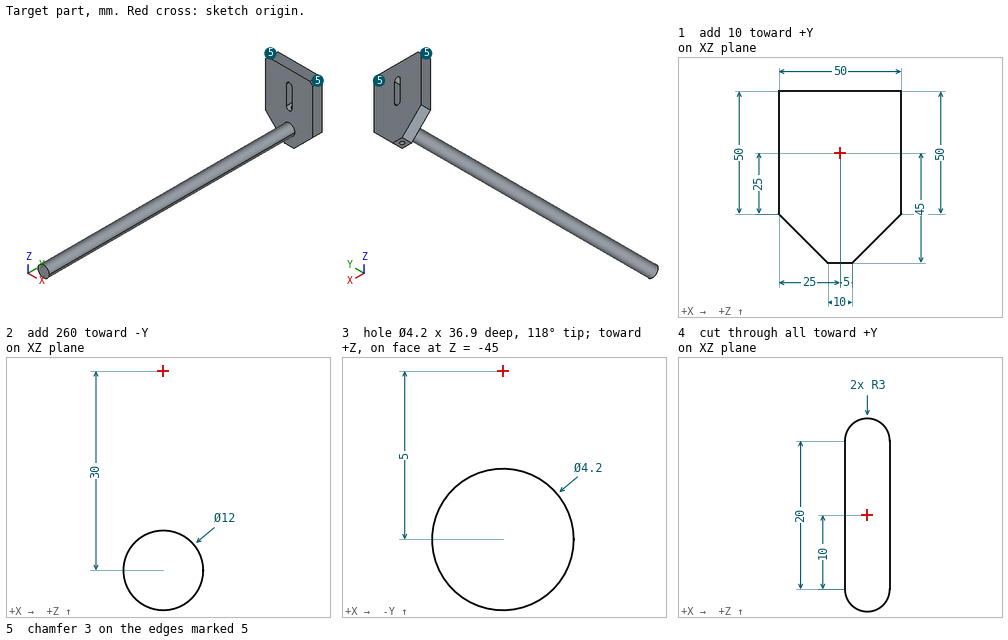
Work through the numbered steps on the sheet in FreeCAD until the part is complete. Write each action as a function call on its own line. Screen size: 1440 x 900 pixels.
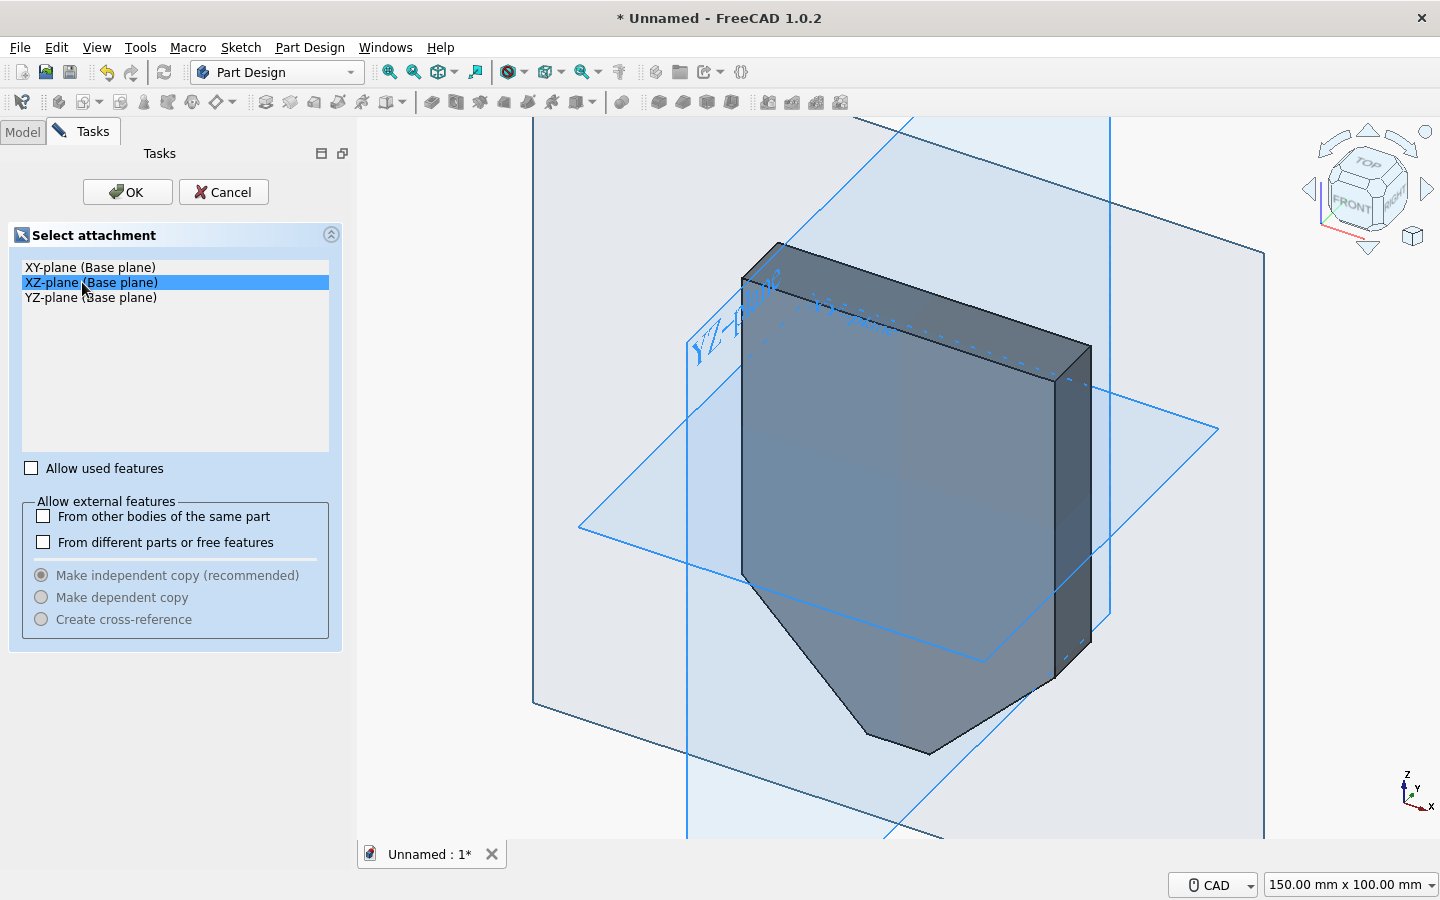
click(128, 192)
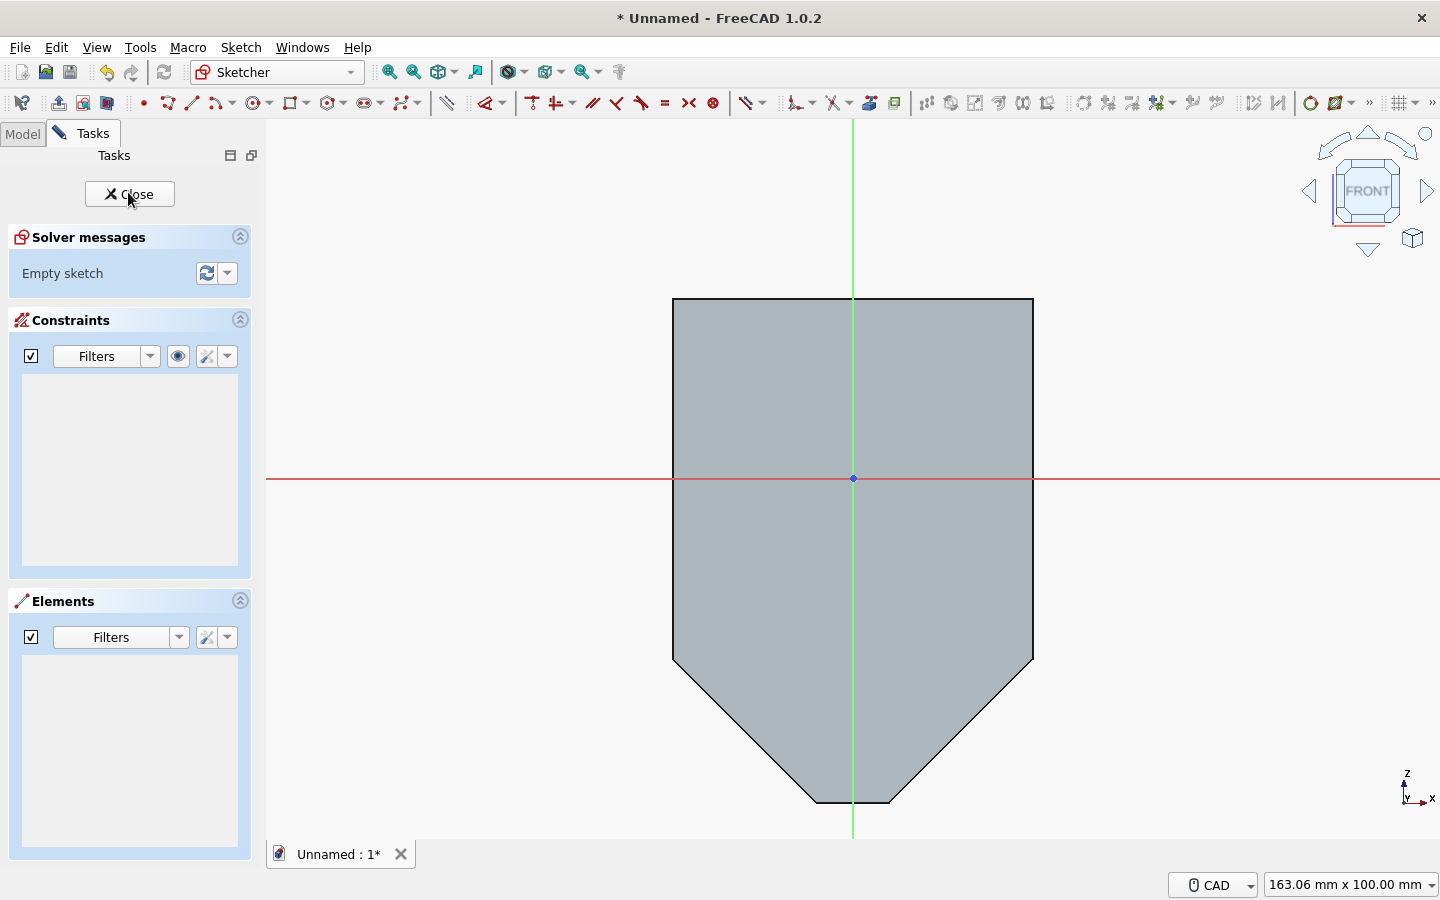
scroll(870, 750, up, 8)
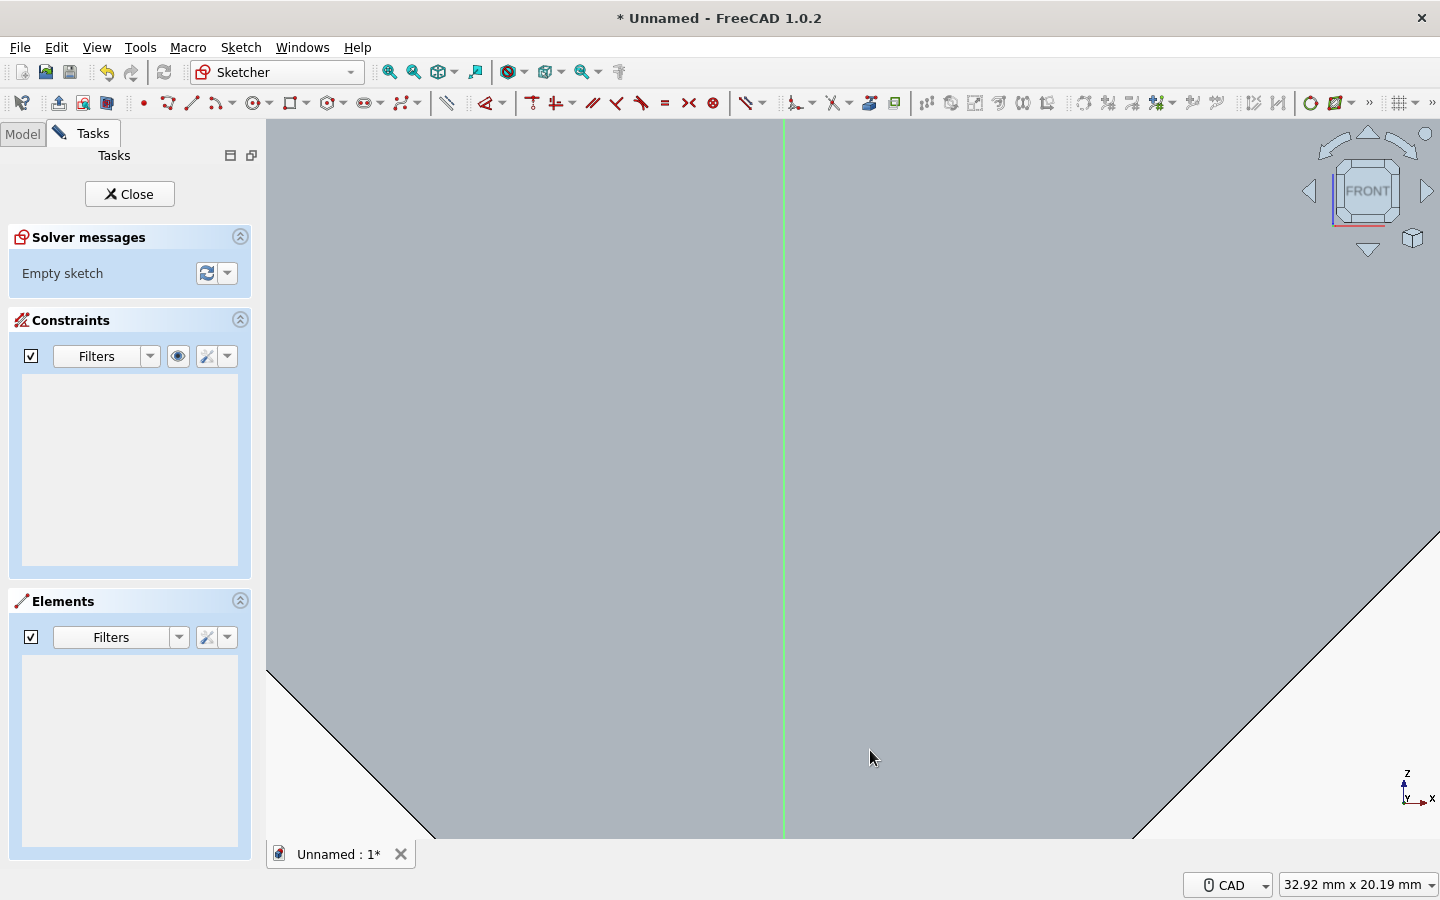
click(254, 104)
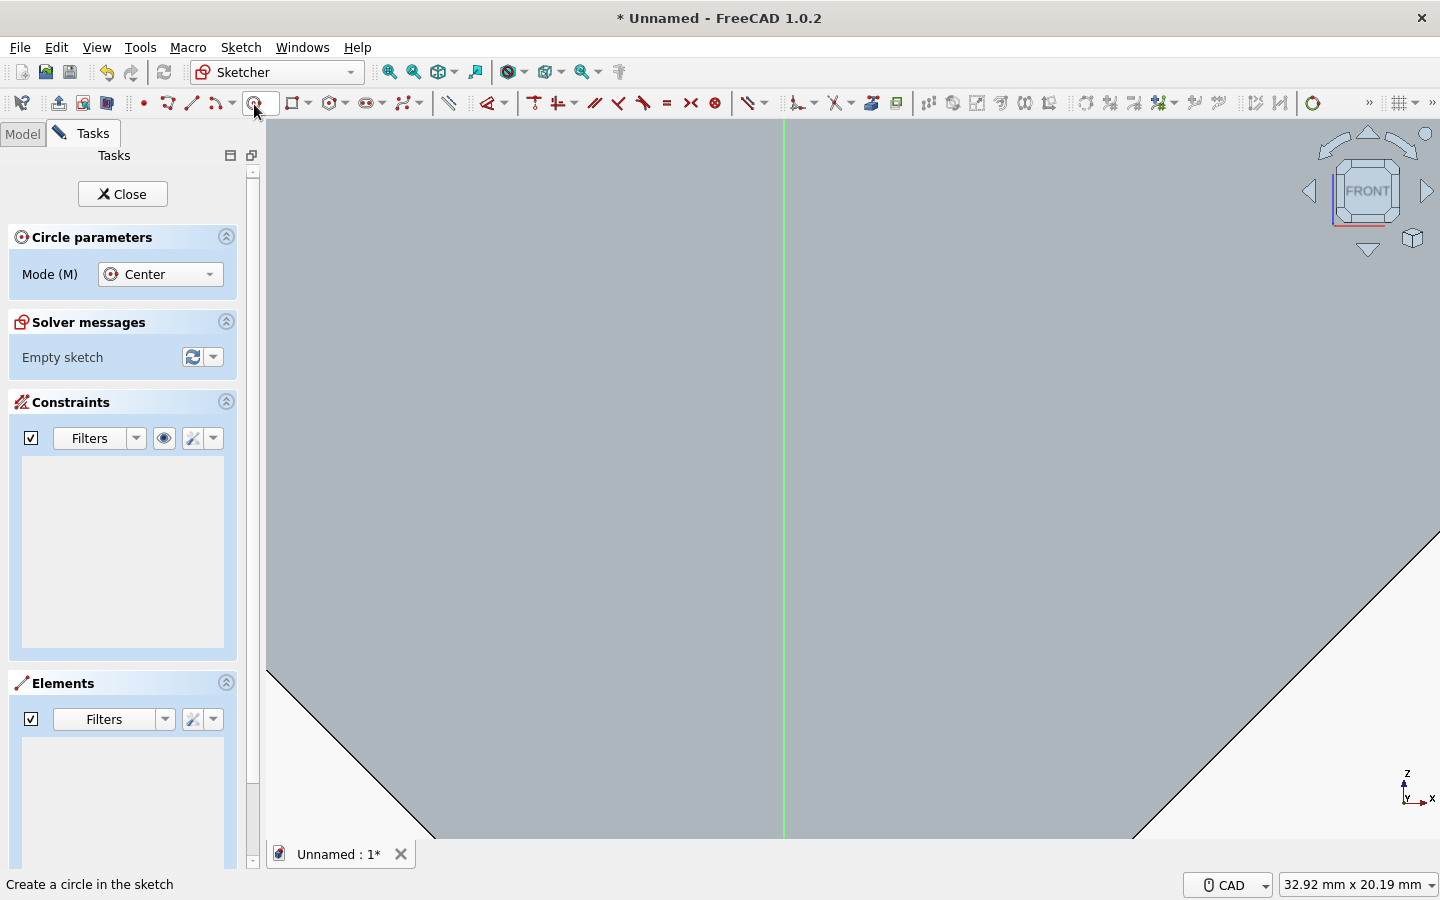
click(784, 474)
move(935, 323)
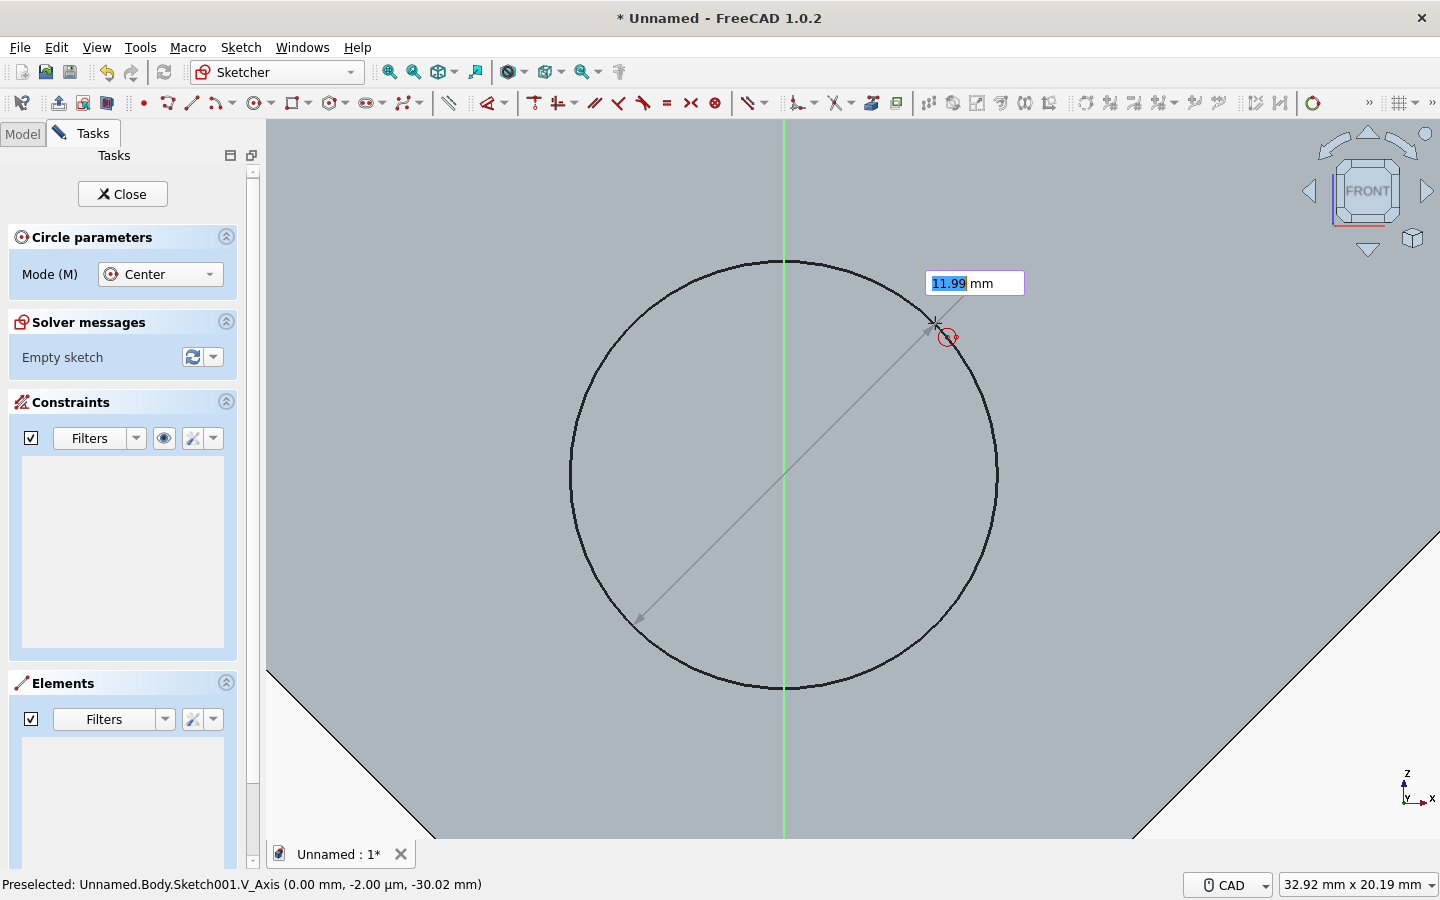
text(12)
key(Return)
key(Escape)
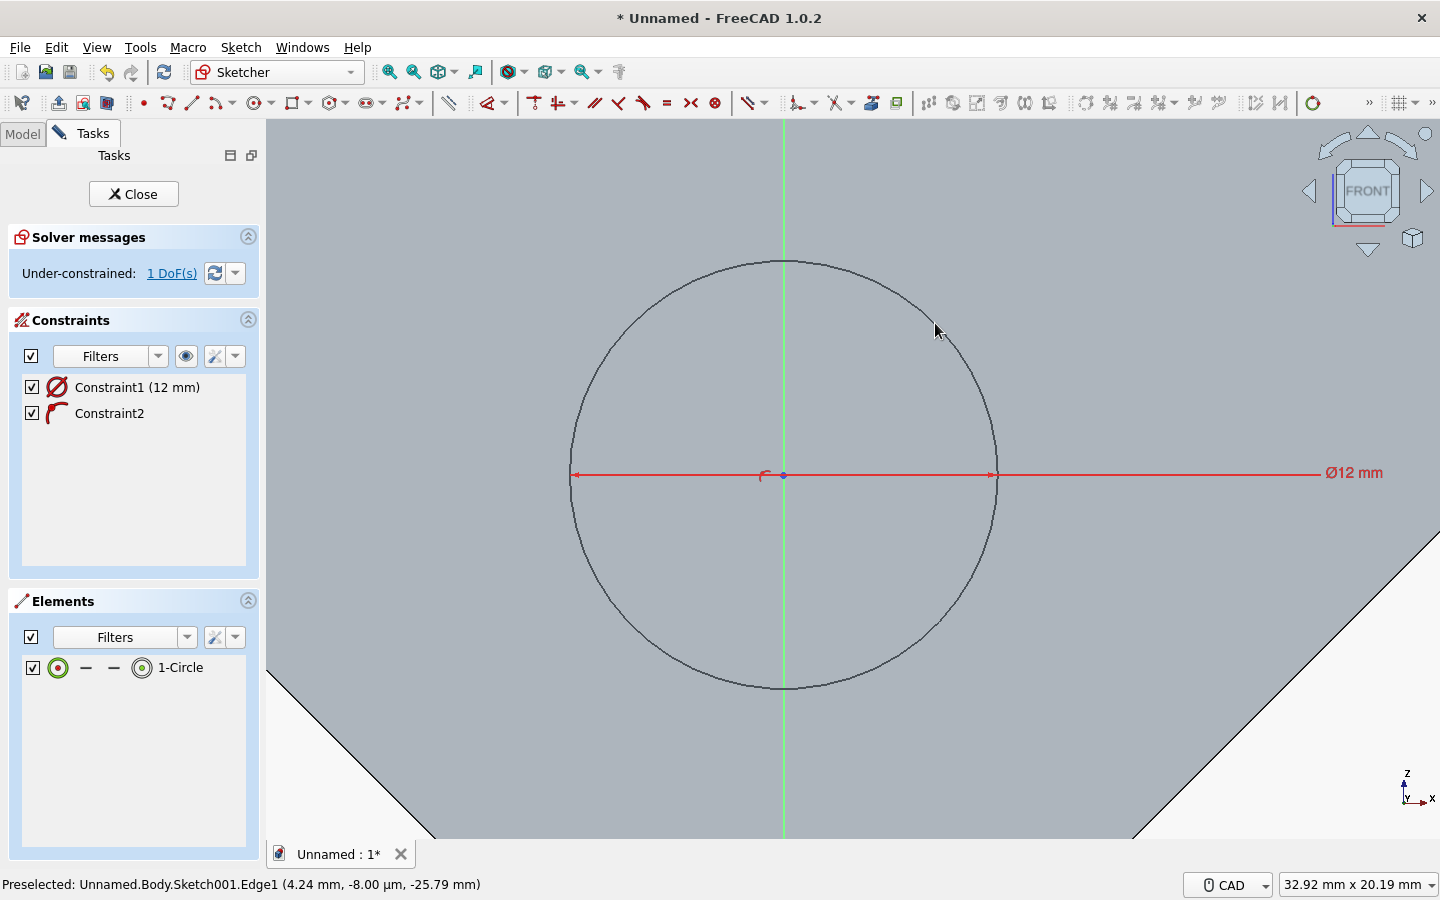
click(488, 104)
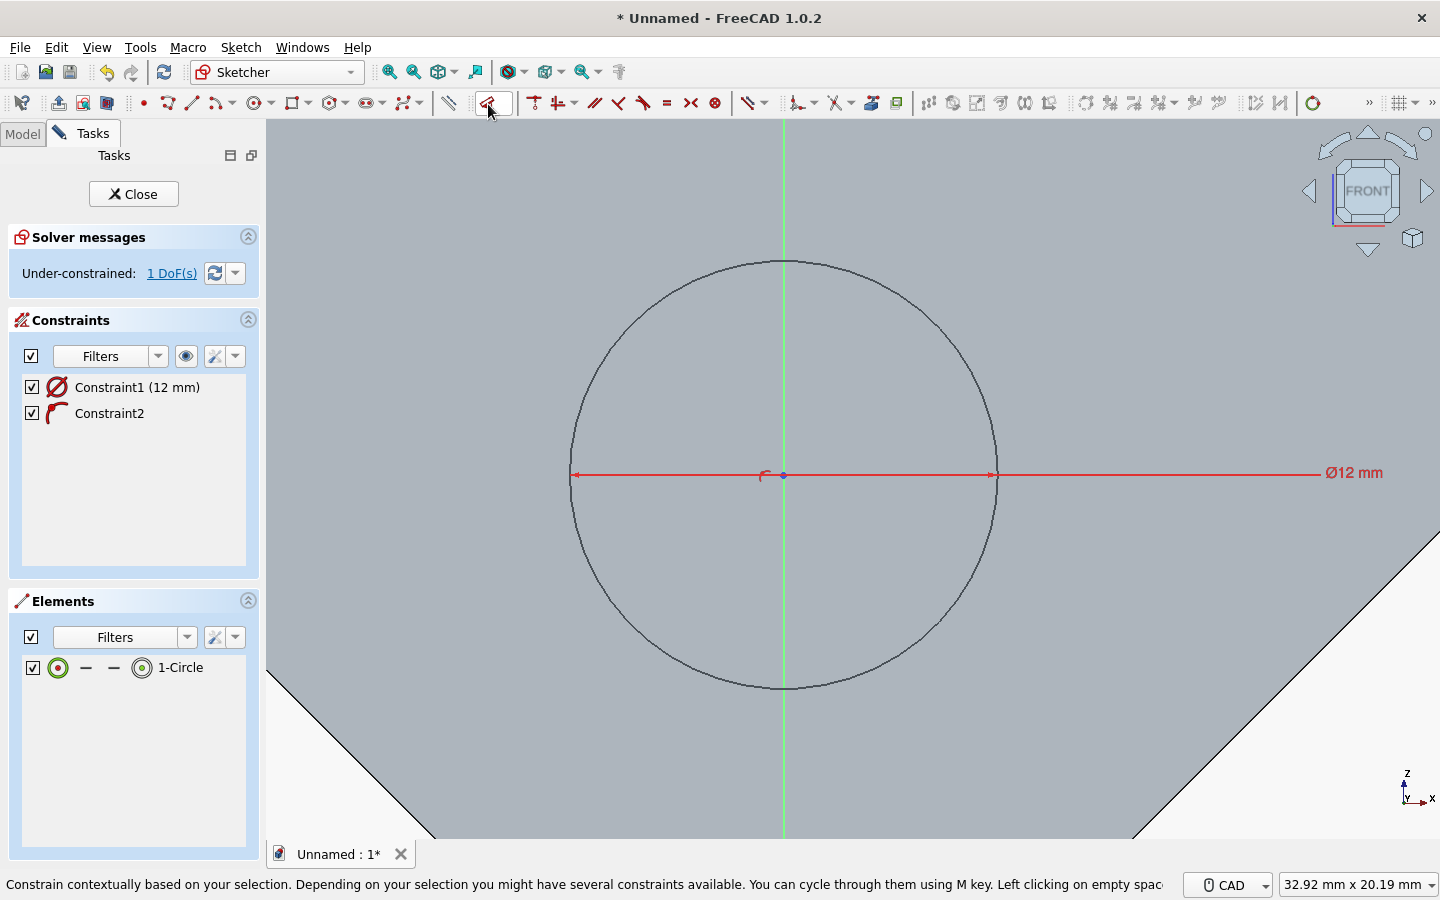
click(784, 475)
click(818, 311)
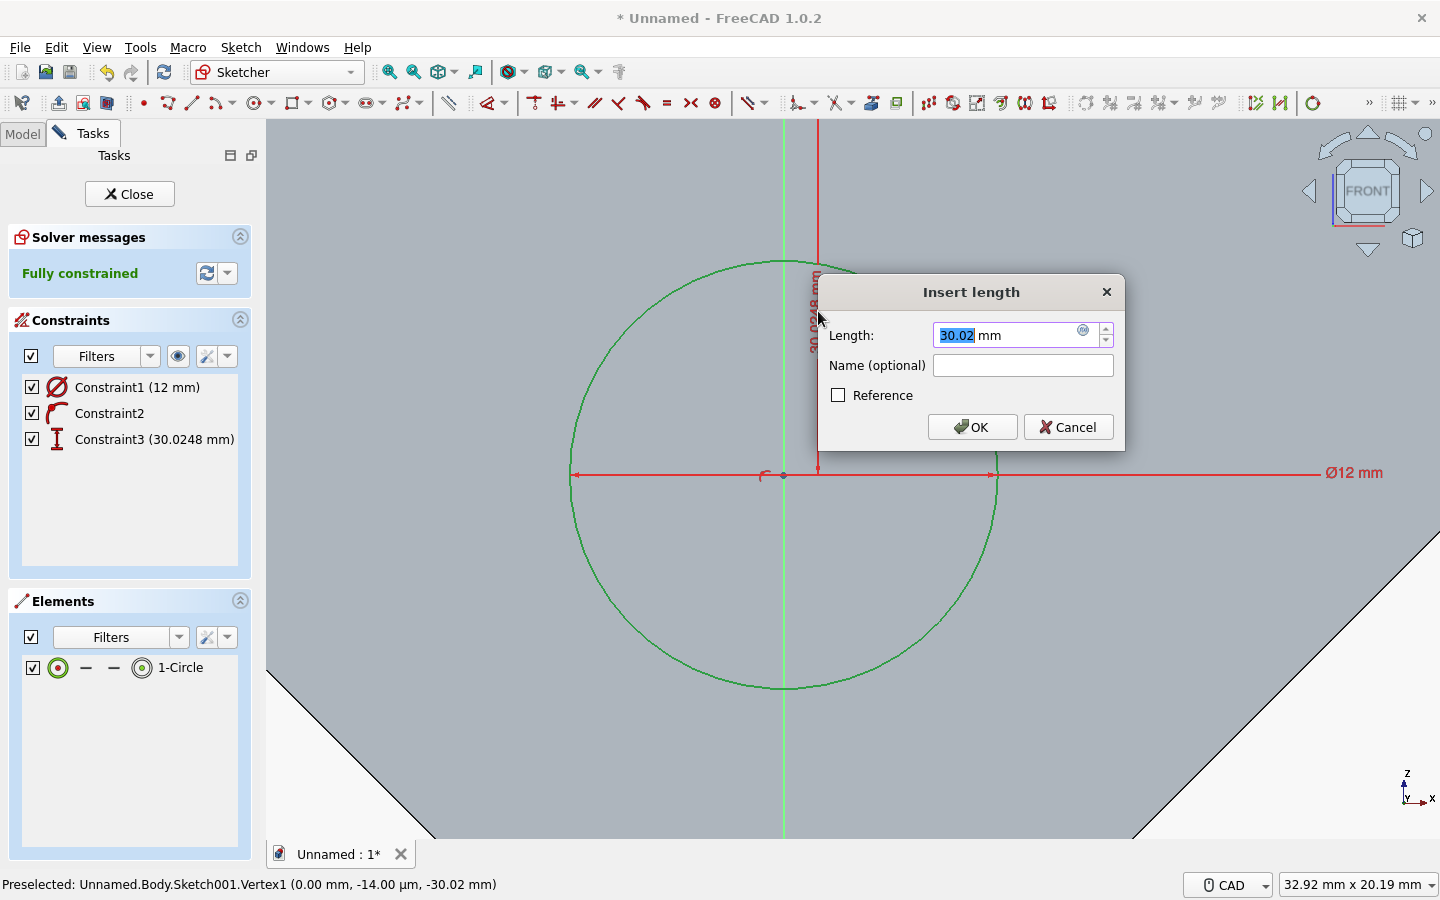
text(30)
key(Return)
key(Escape)